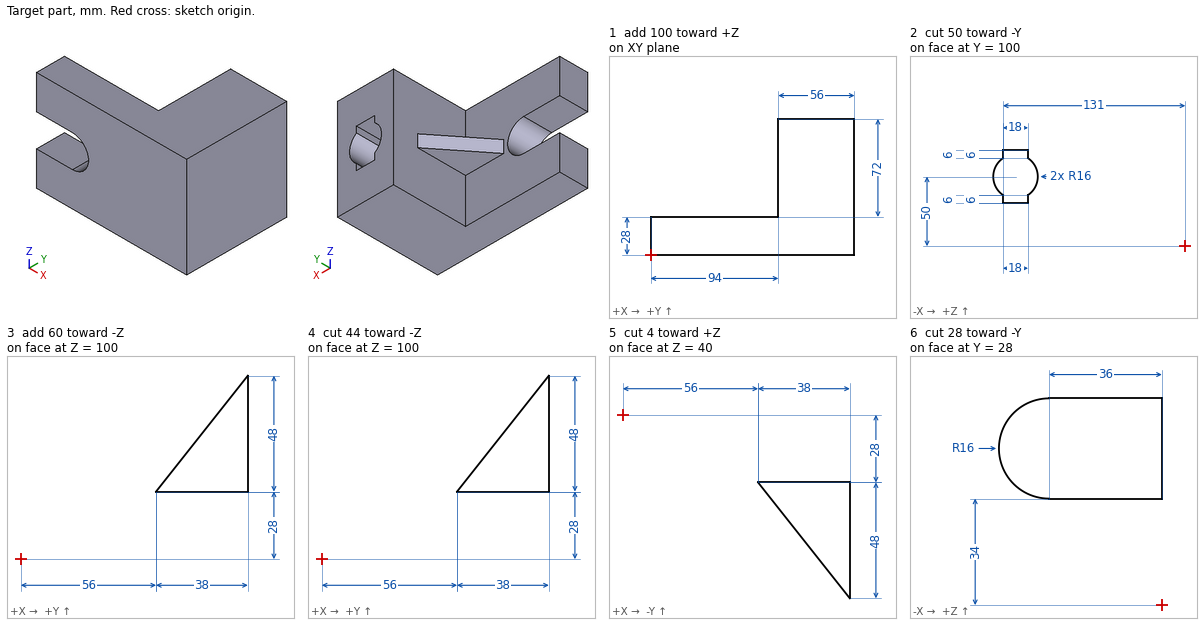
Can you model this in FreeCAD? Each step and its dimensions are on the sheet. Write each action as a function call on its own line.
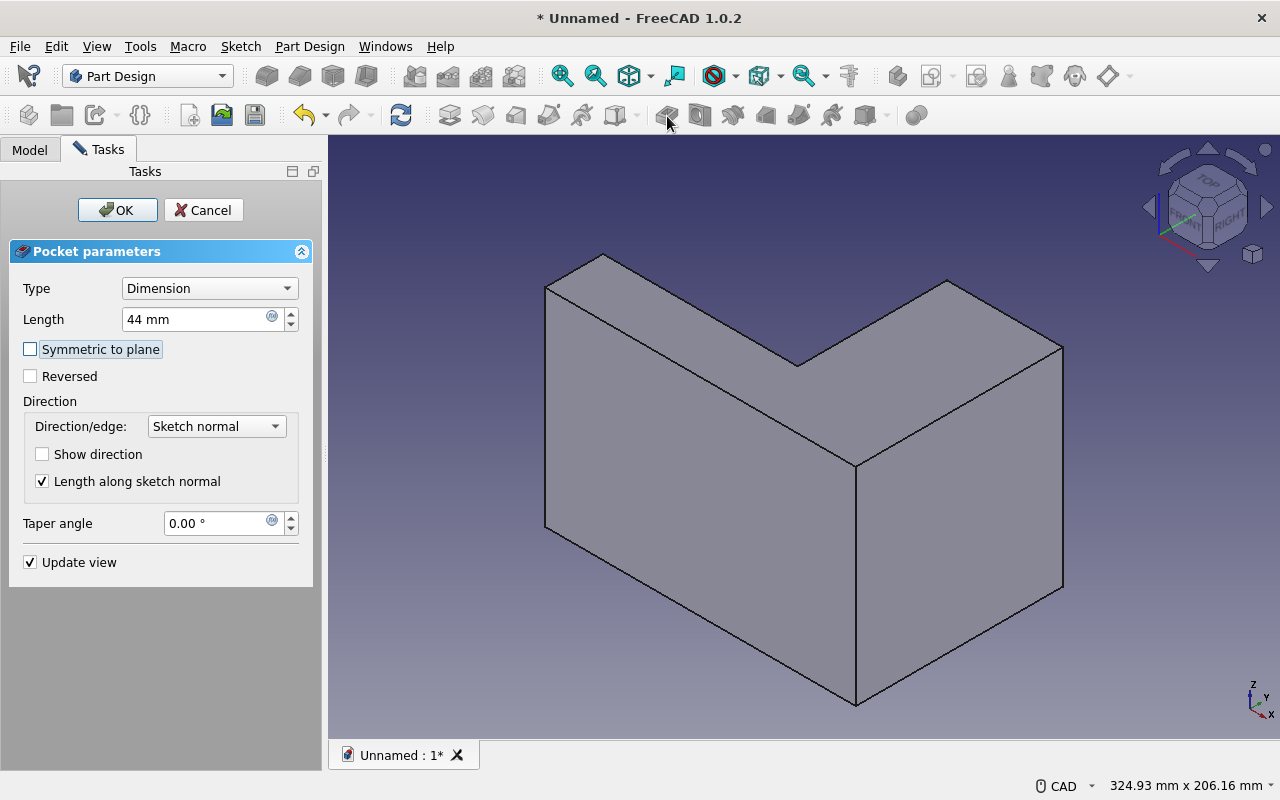
click(118, 210)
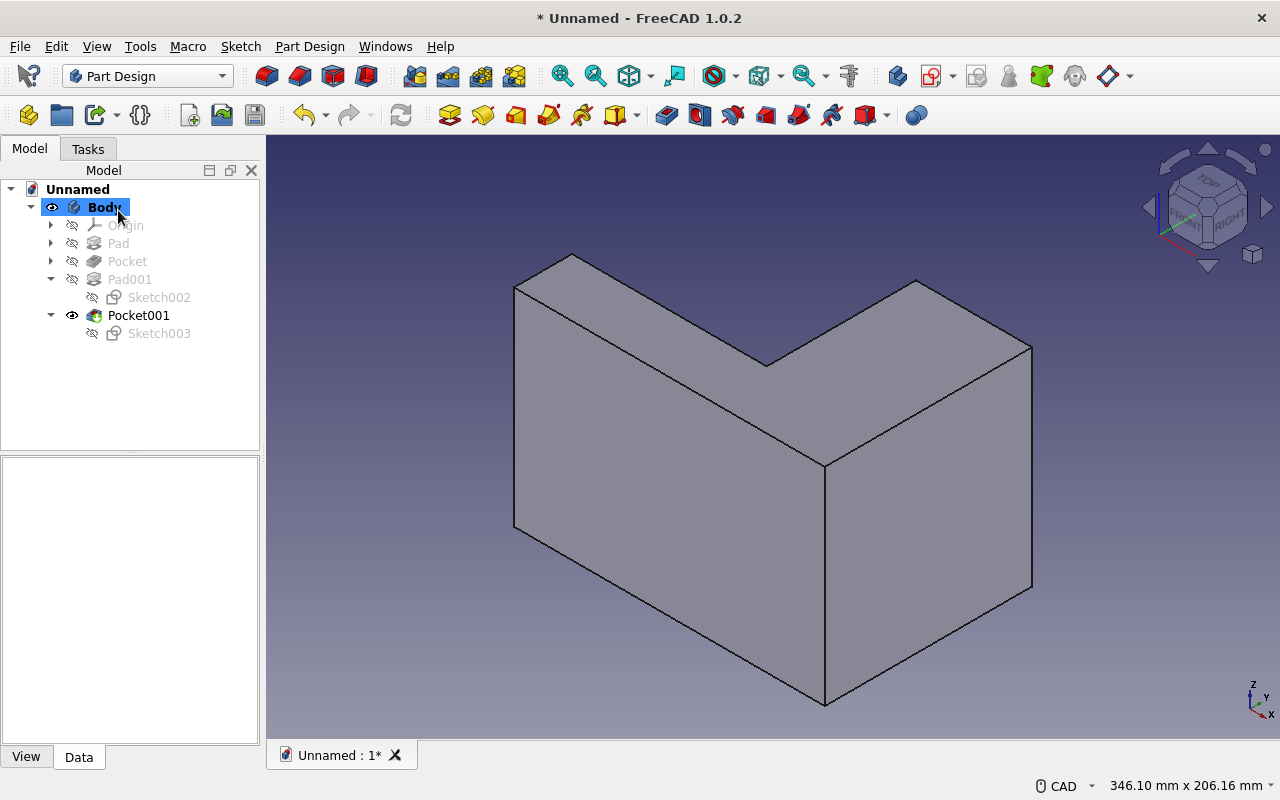
key(5)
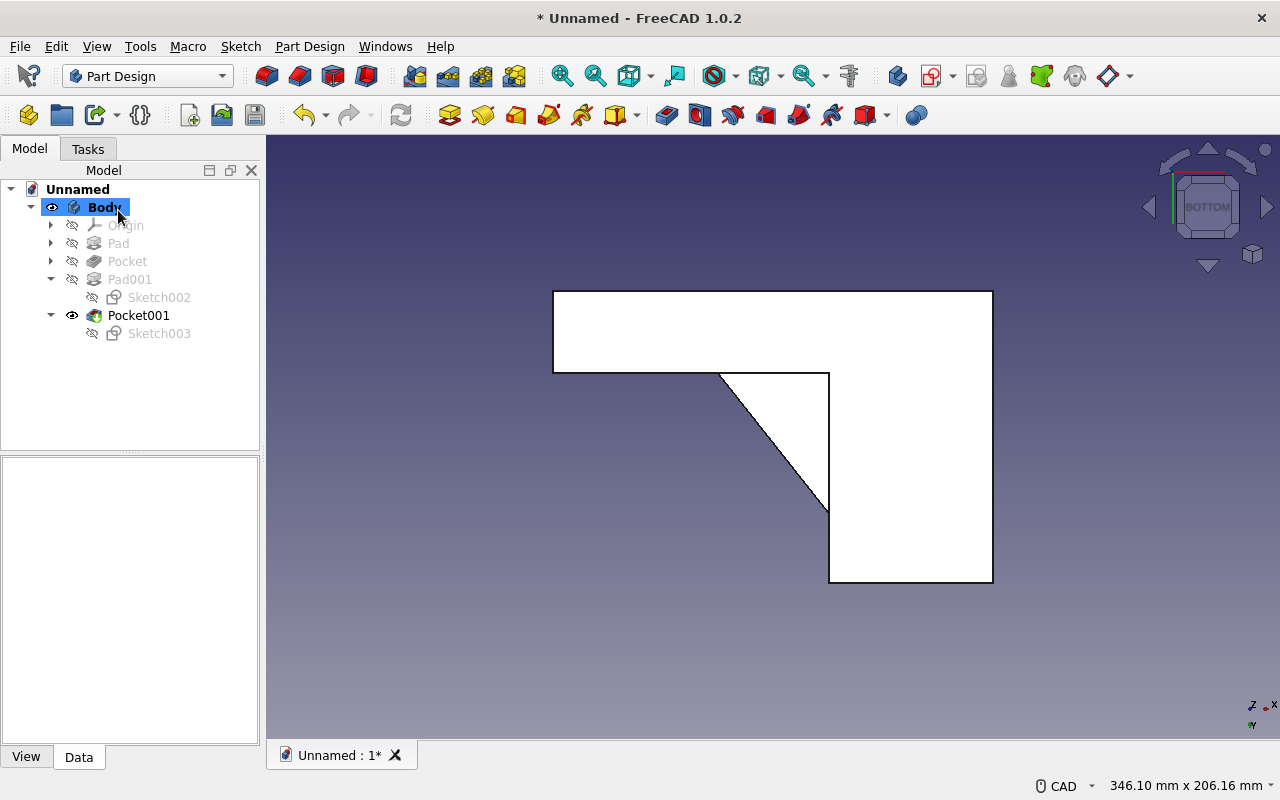
click(789, 402)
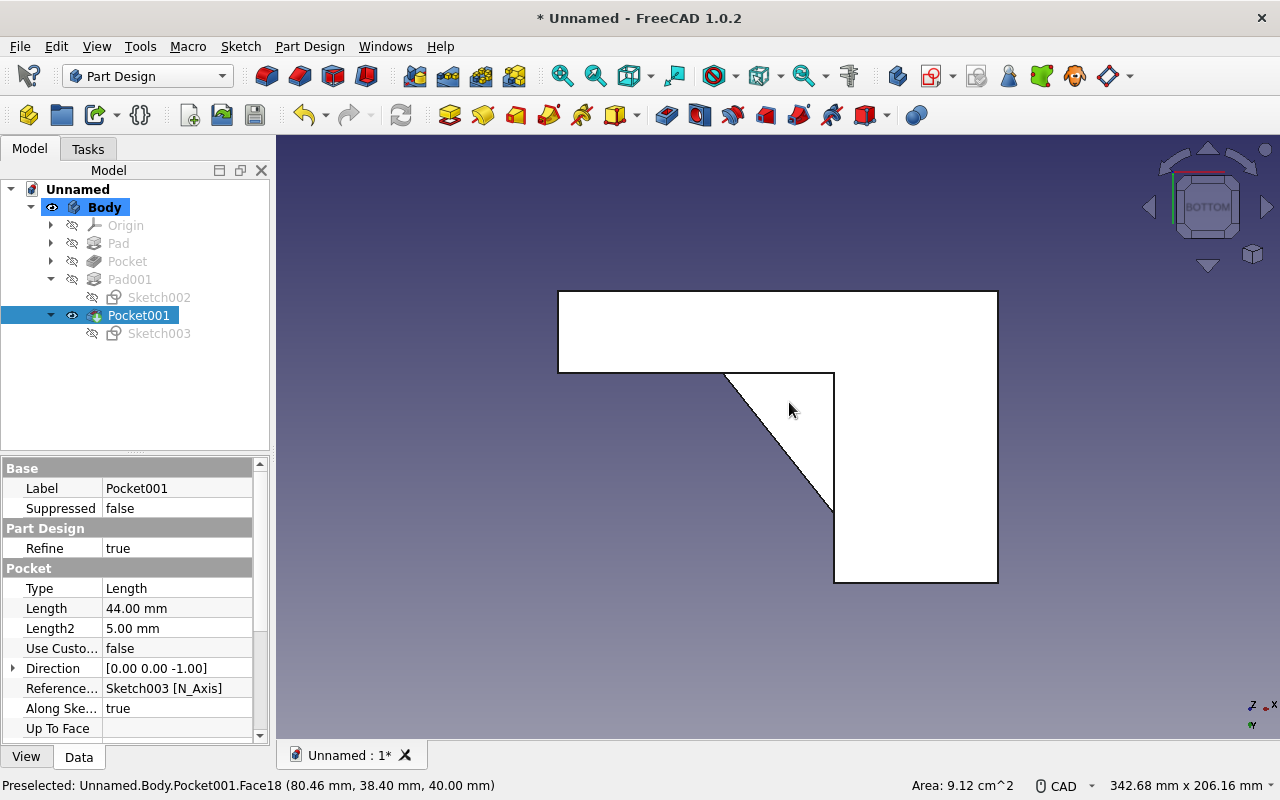
click(930, 76)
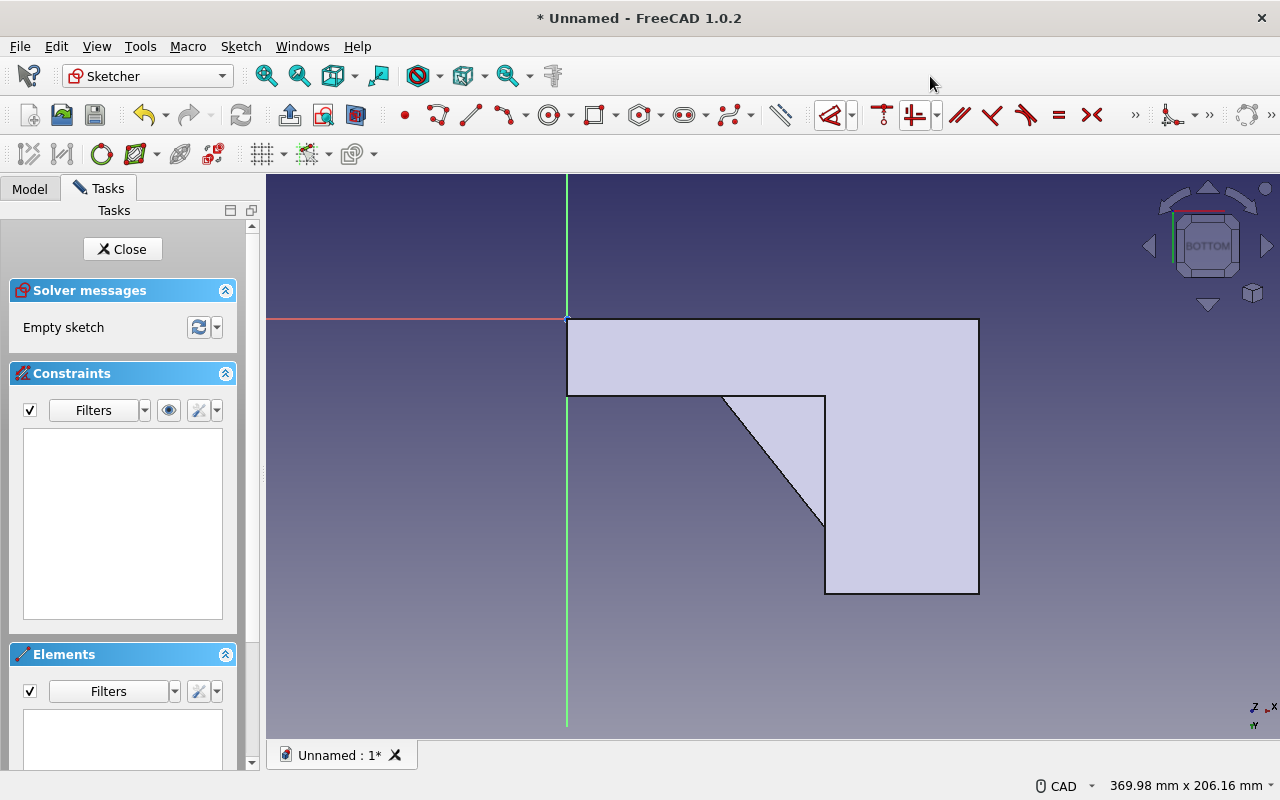
scroll(686, 384, up, 3)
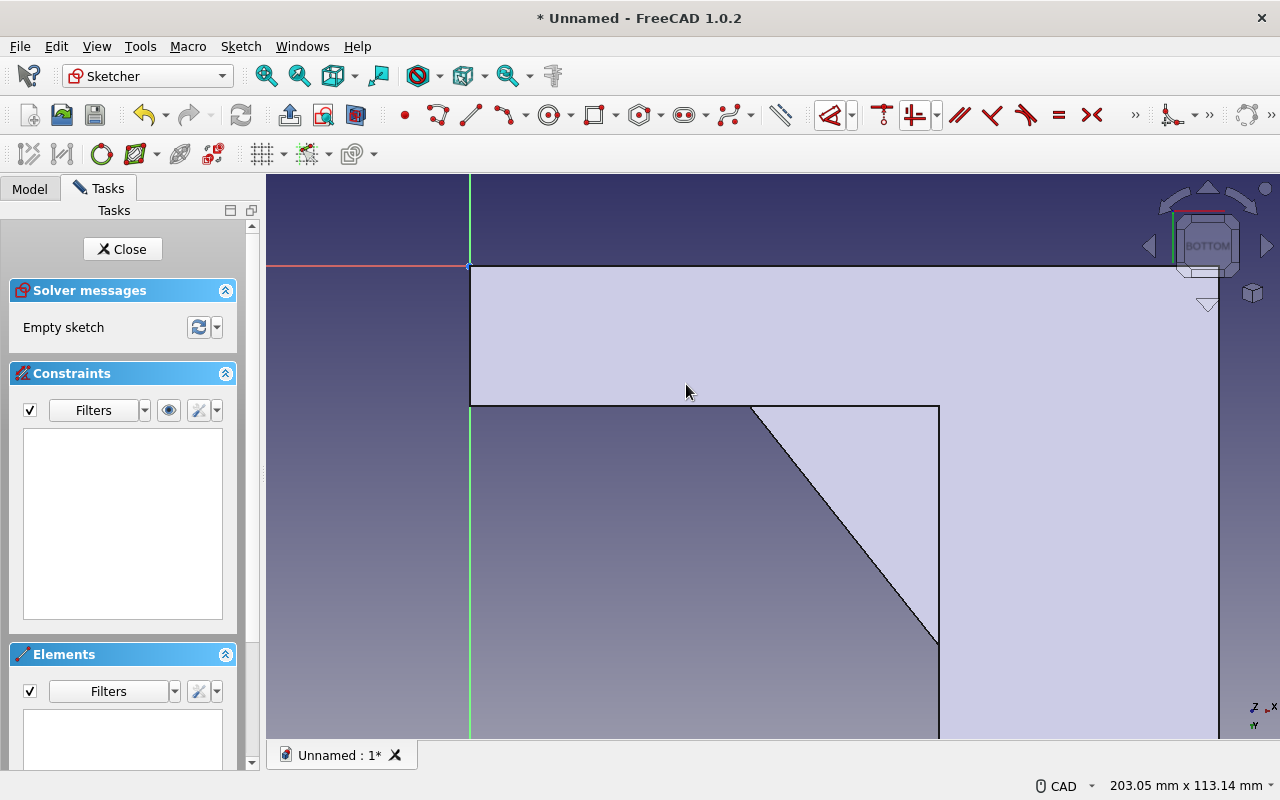
click(438, 116)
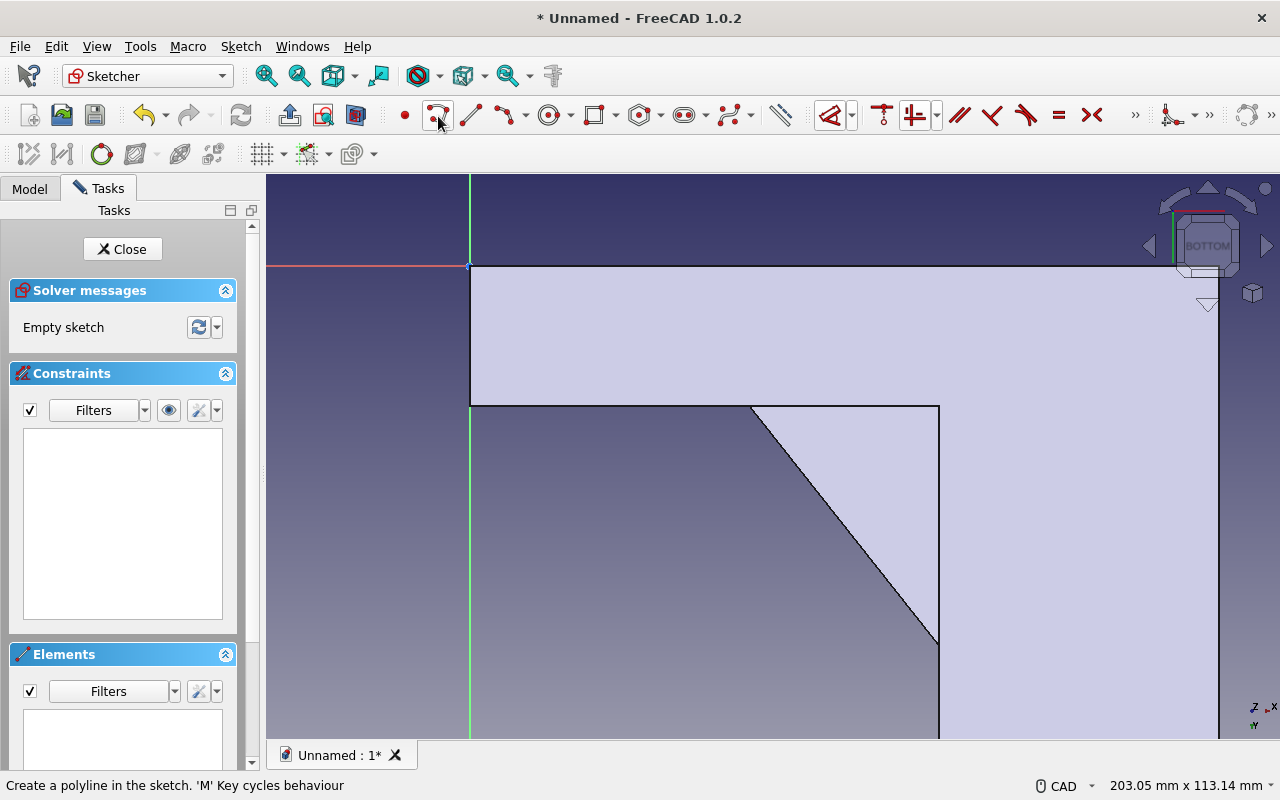
click(749, 406)
click(939, 646)
click(939, 406)
click(749, 407)
key(Escape)
key(Escape)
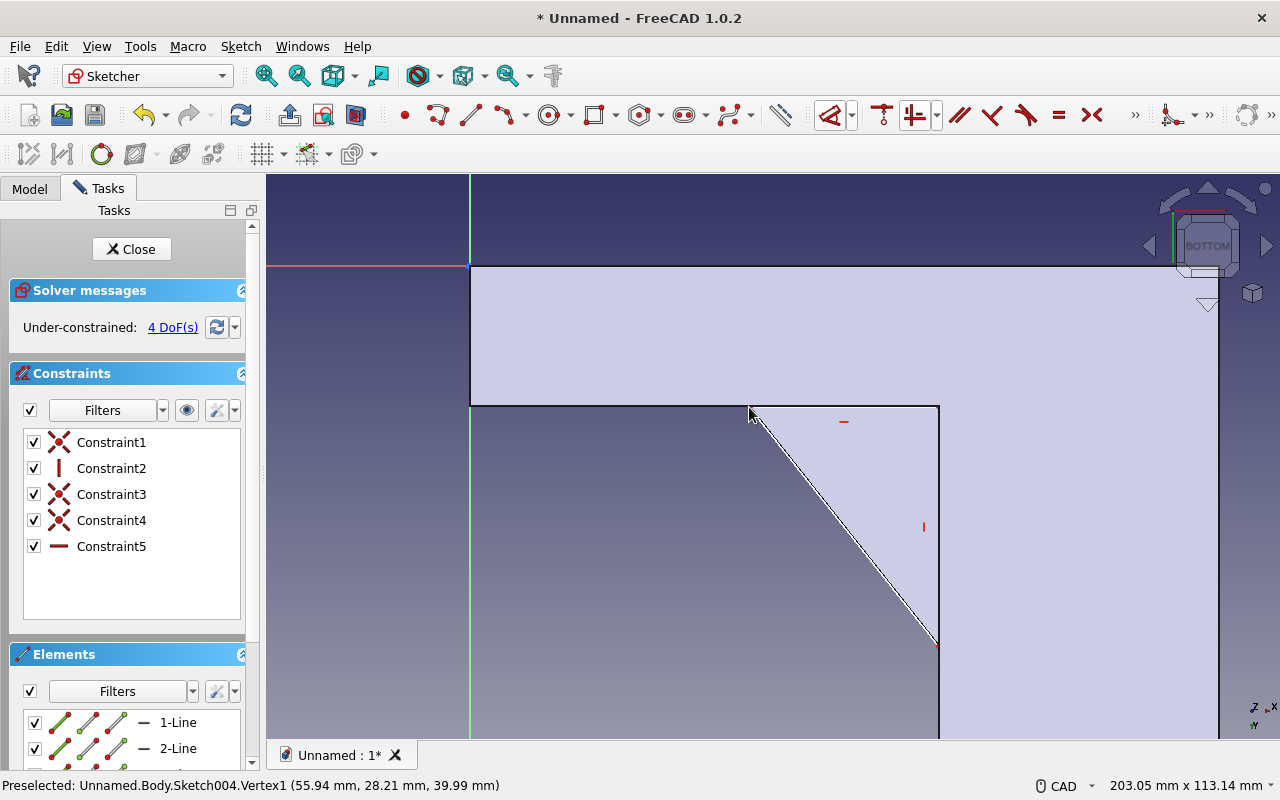
click(939, 575)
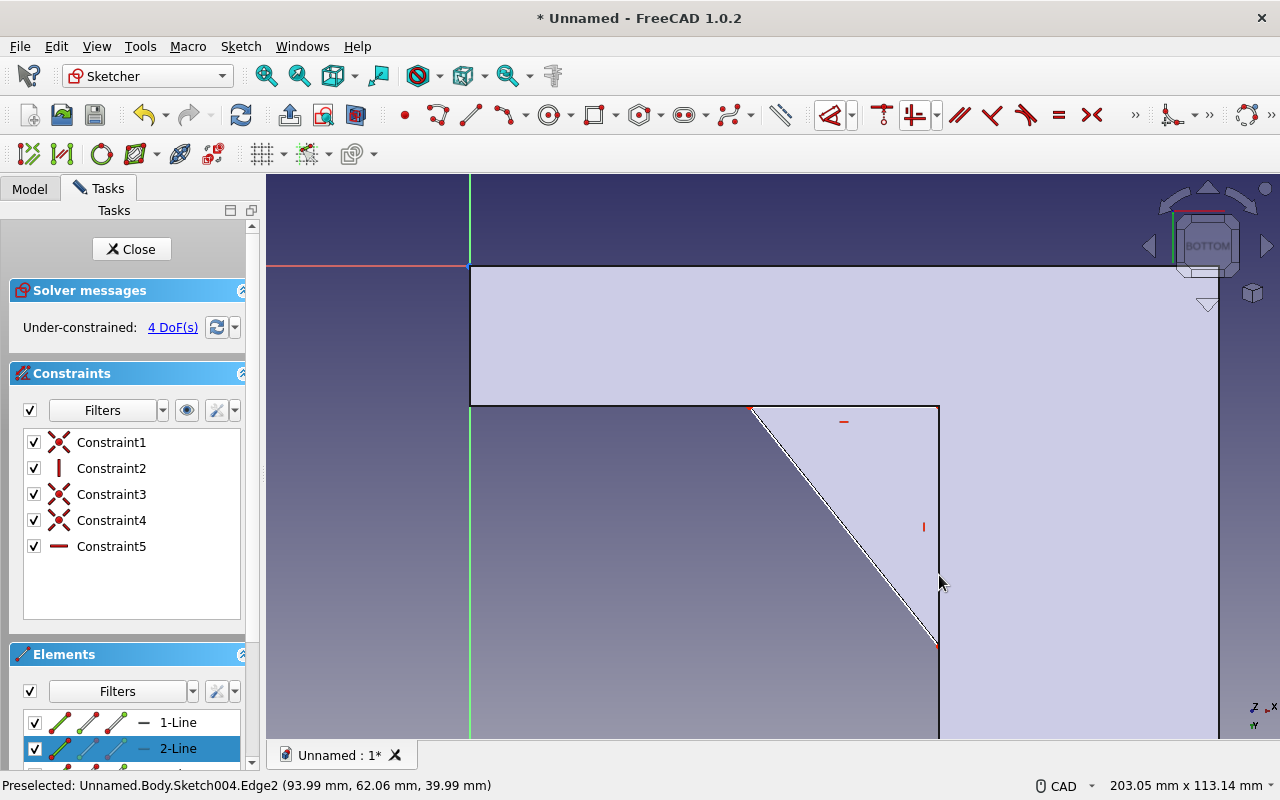
click(852, 116)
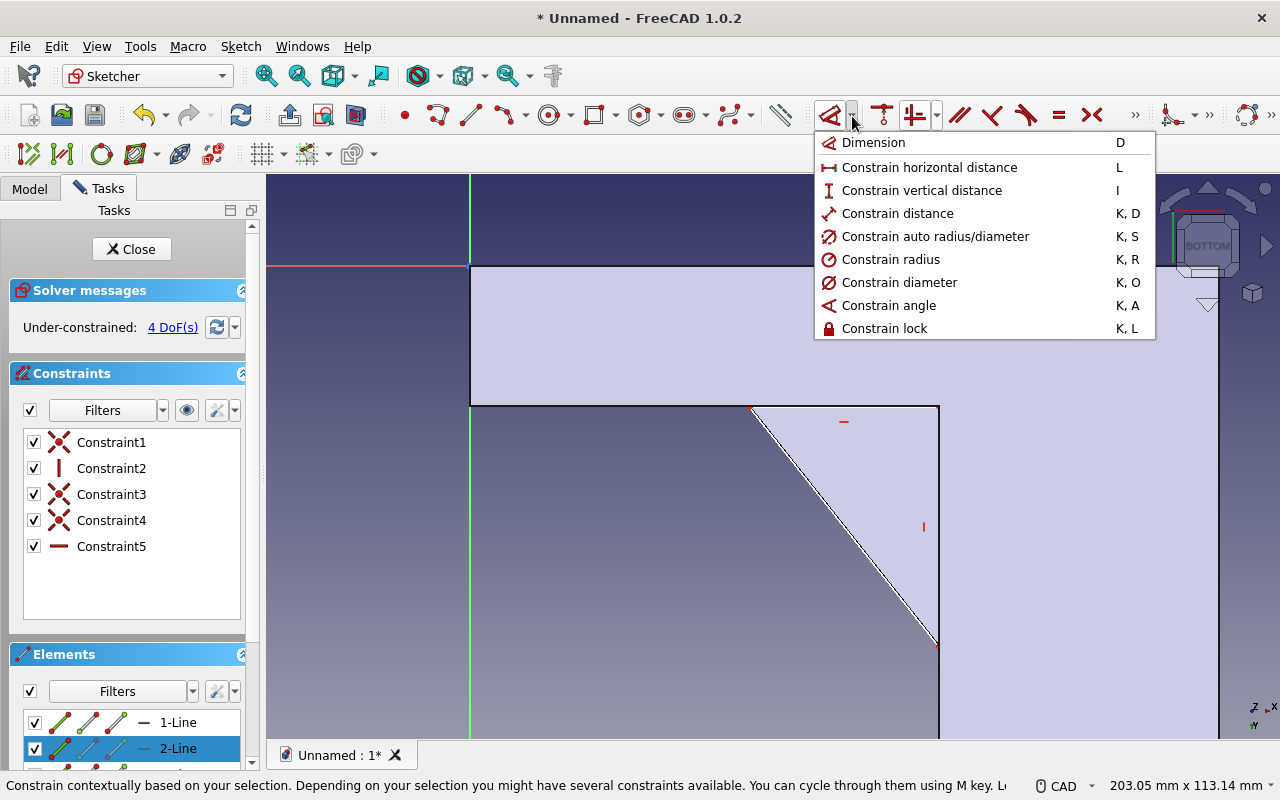
click(985, 190)